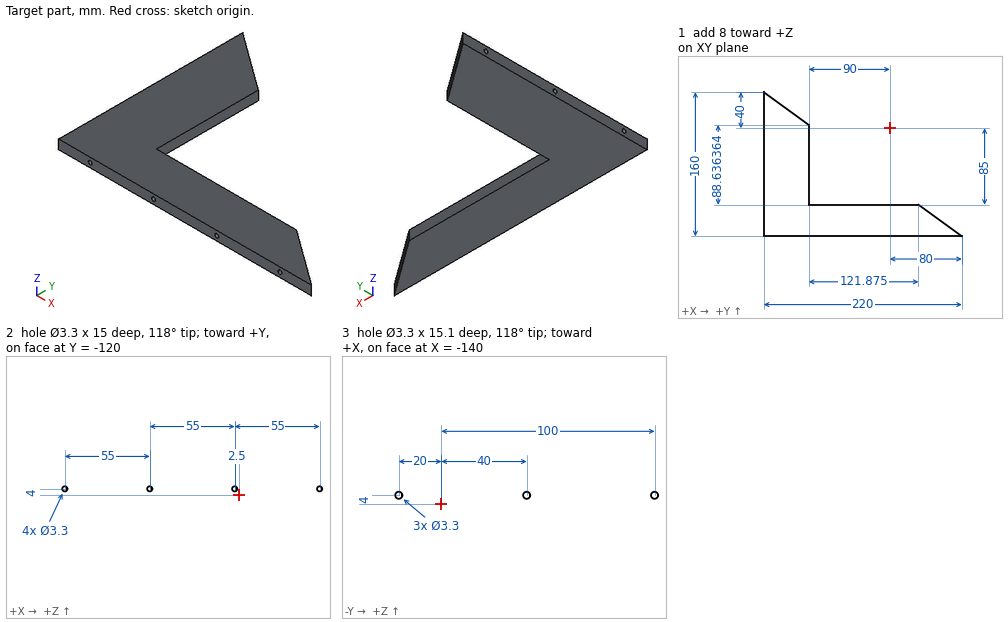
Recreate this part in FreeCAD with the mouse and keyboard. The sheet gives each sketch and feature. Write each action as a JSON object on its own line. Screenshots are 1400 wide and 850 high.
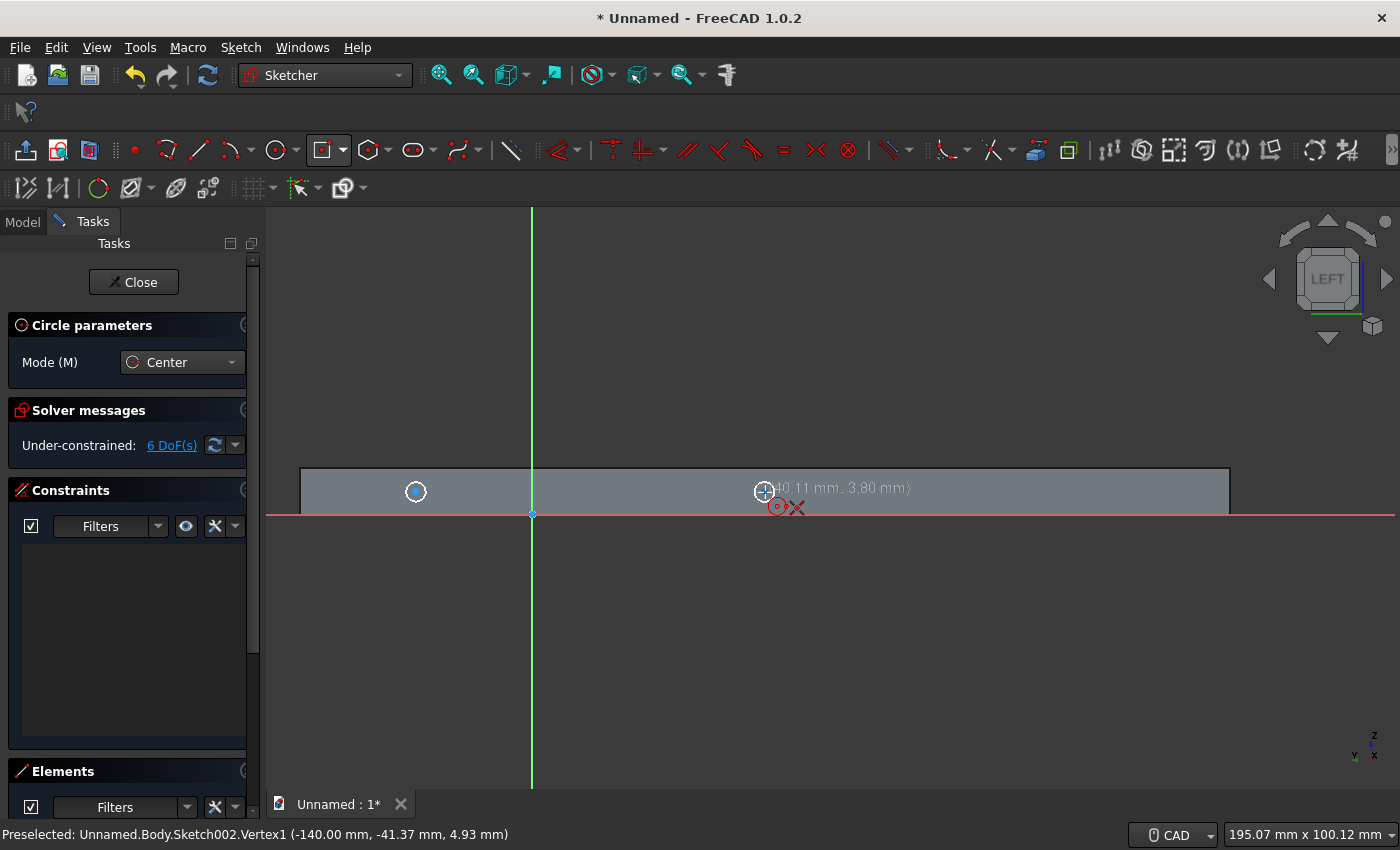
{"action": "scroll", "coordinate": [1113, 492], "scroll_direction": "up", "scroll_amount": 5}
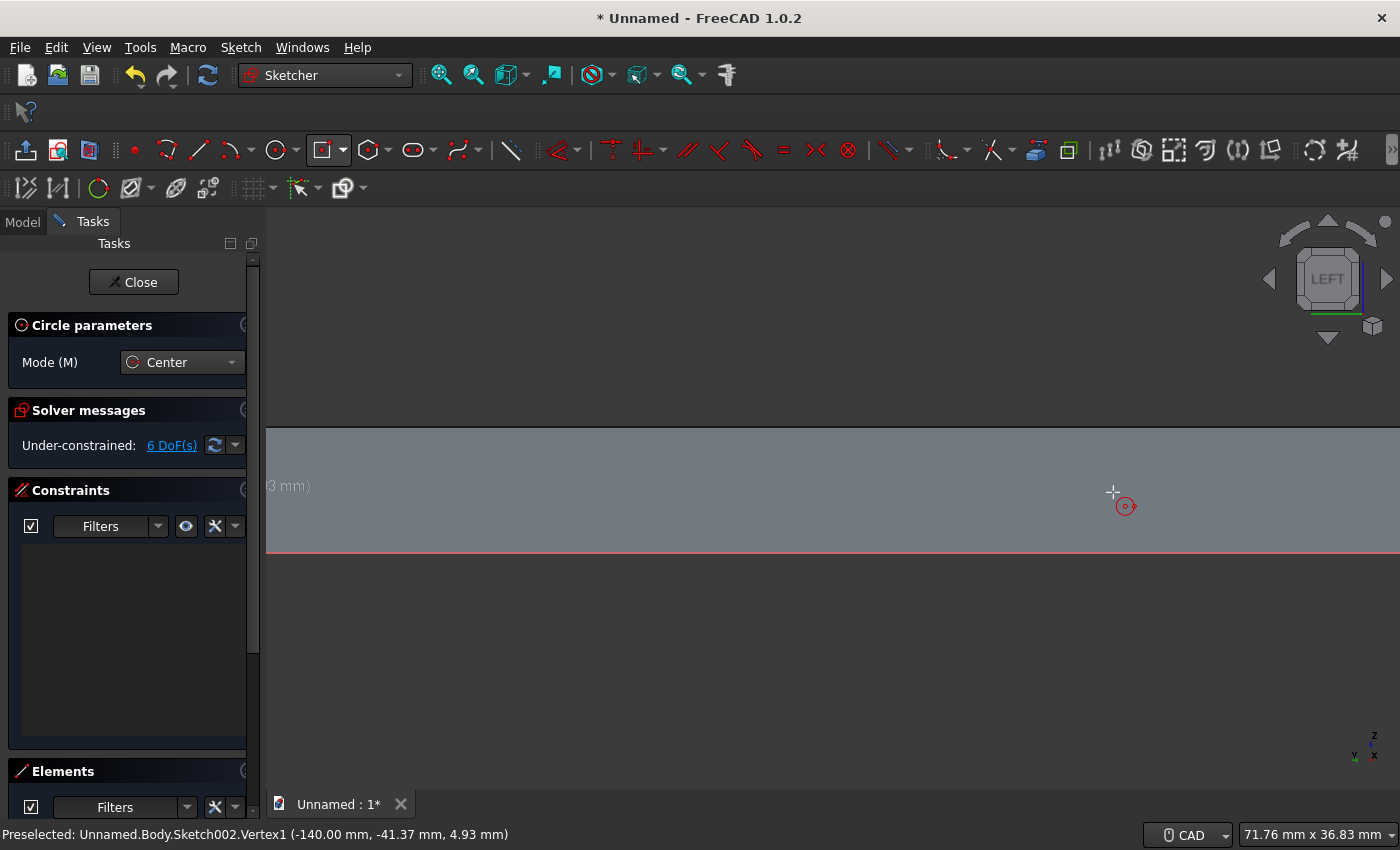
{"action": "left_click", "coordinate": [1113, 490]}
{"action": "left_click", "coordinate": [1131, 471]}
{"action": "key", "text": "Escape"}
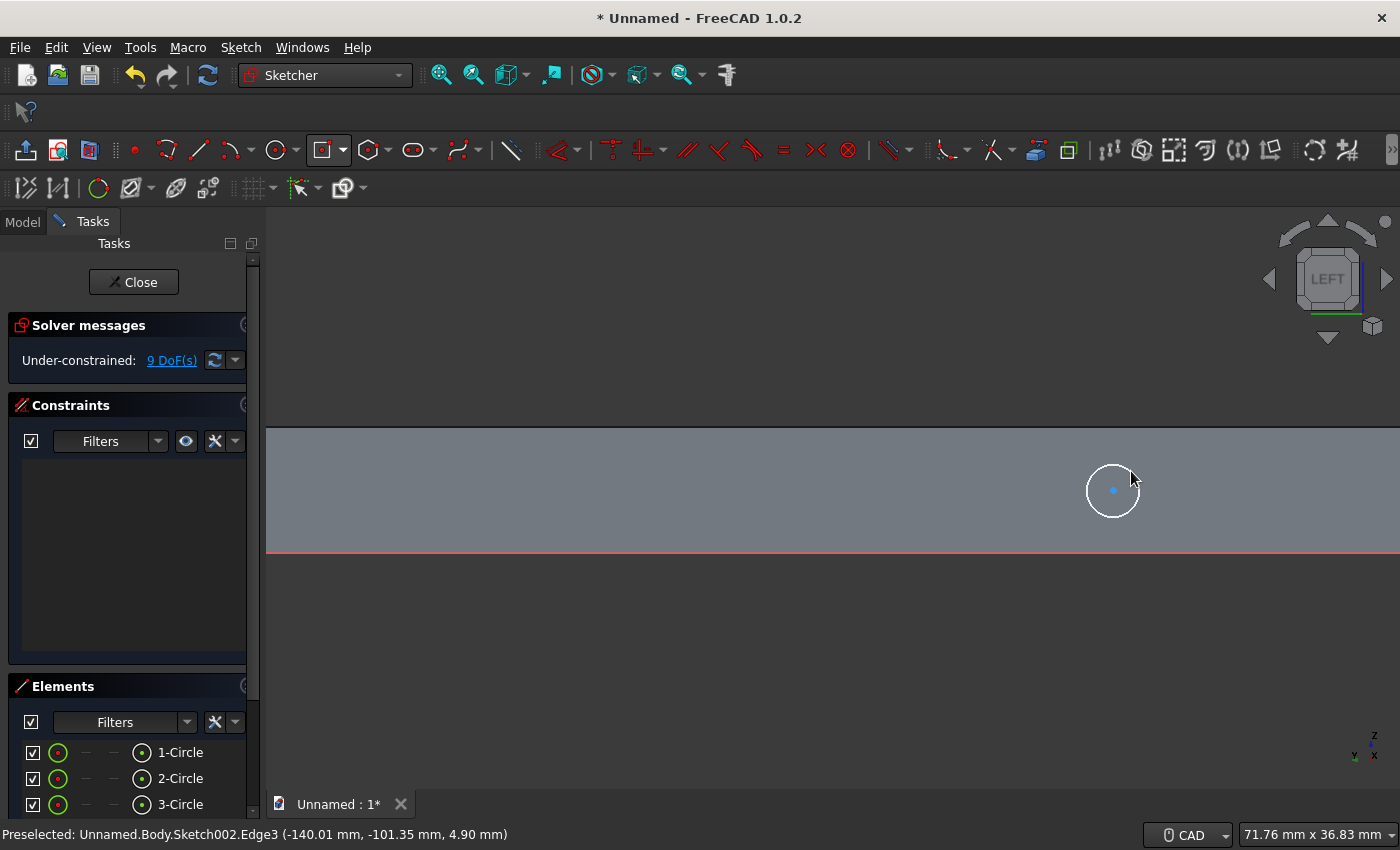
{"action": "scroll", "coordinate": [1114, 492], "scroll_direction": "down", "scroll_amount": 5}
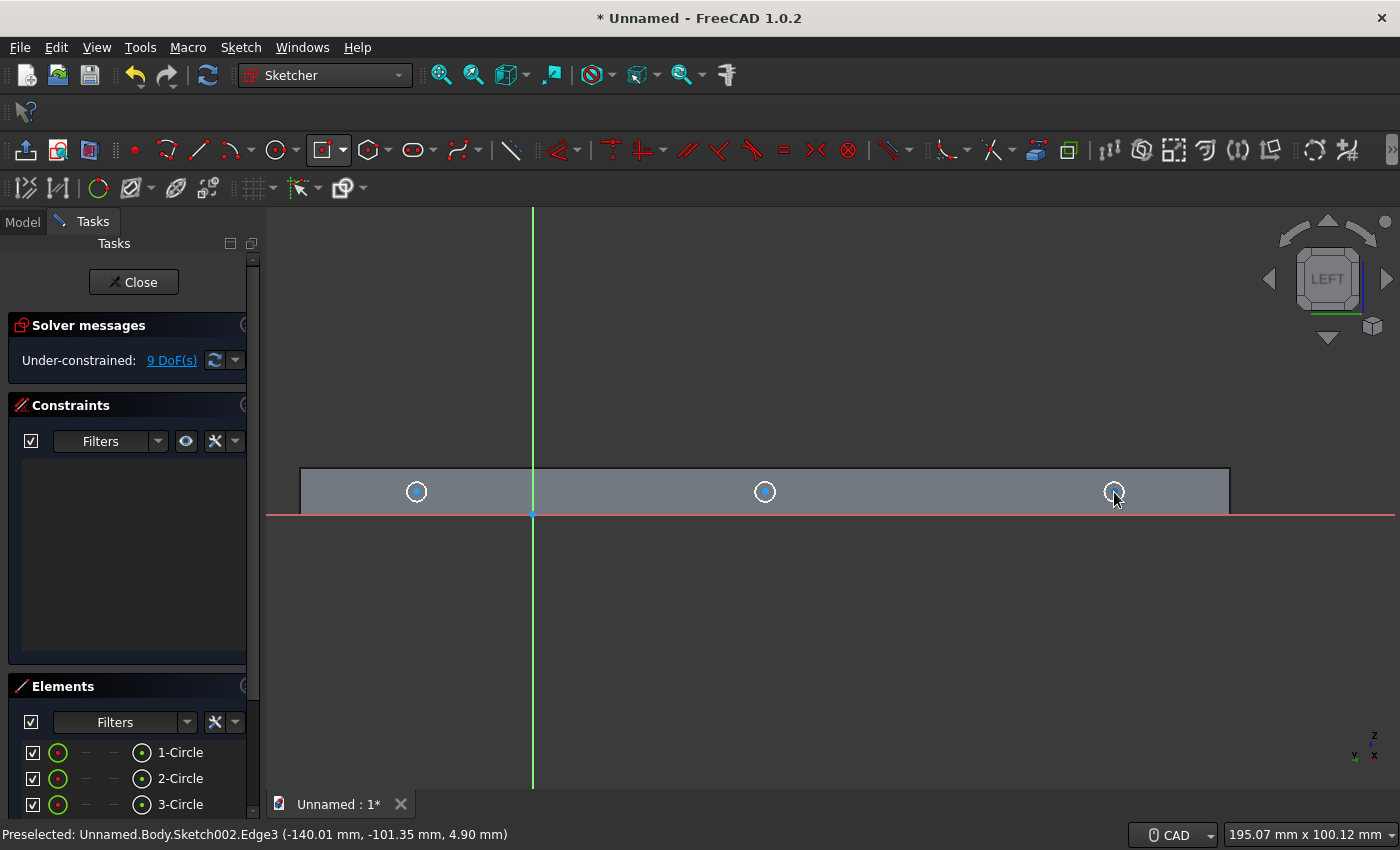
{"action": "scroll", "coordinate": [423, 485], "scroll_direction": "up", "scroll_amount": 2}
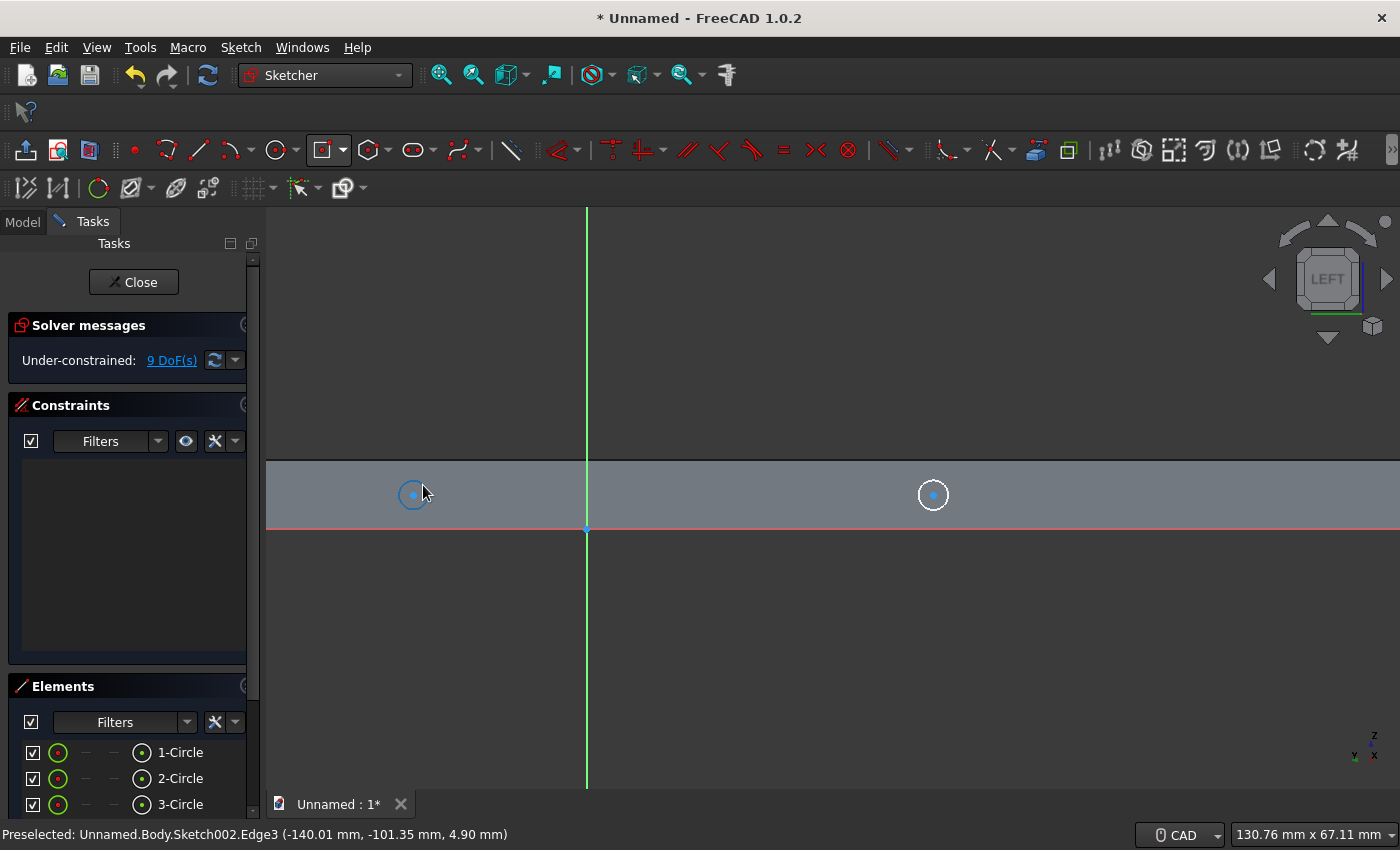
{"action": "left_click", "coordinate": [424, 485]}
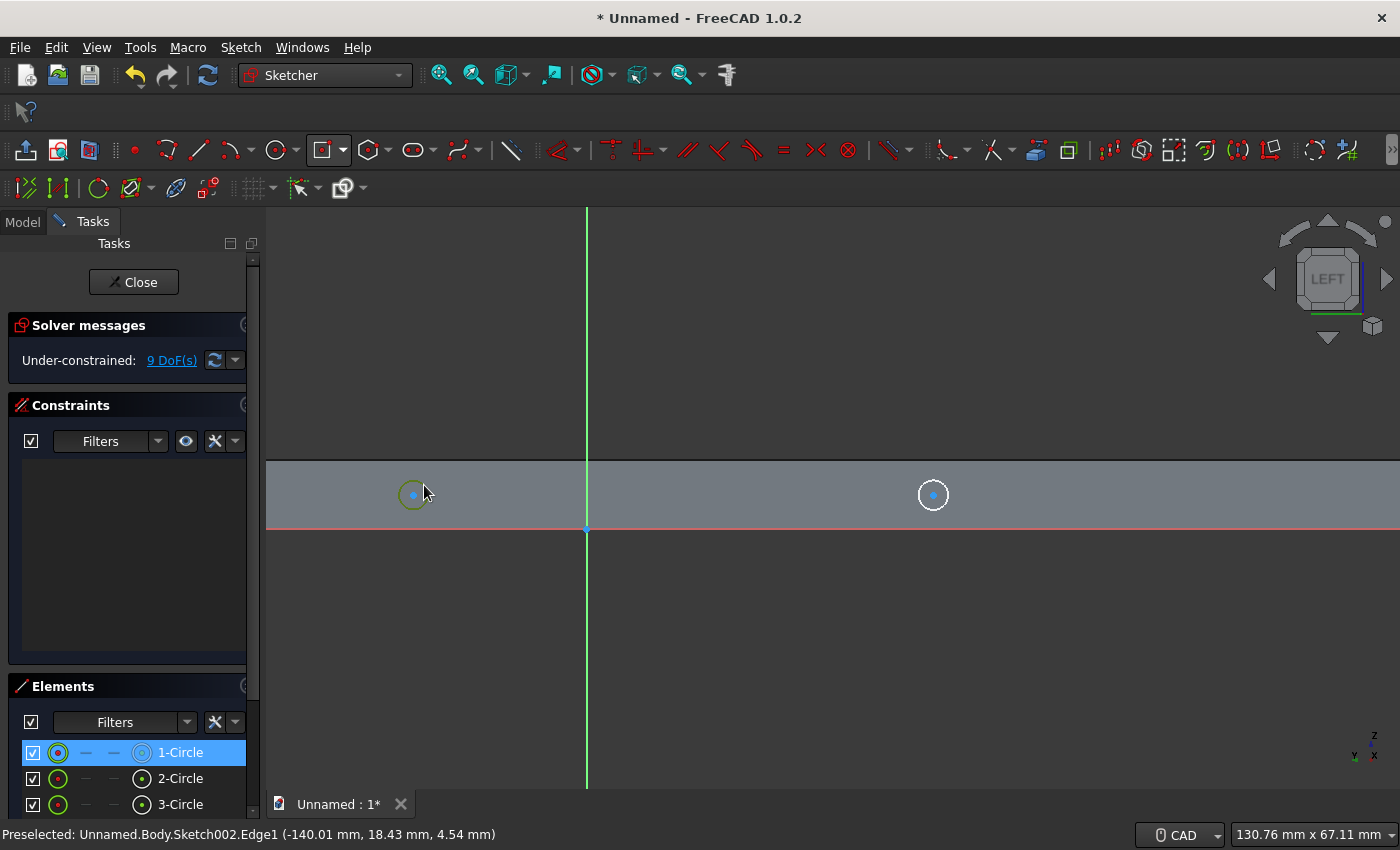
{"action": "left_click", "coordinate": [944, 485]}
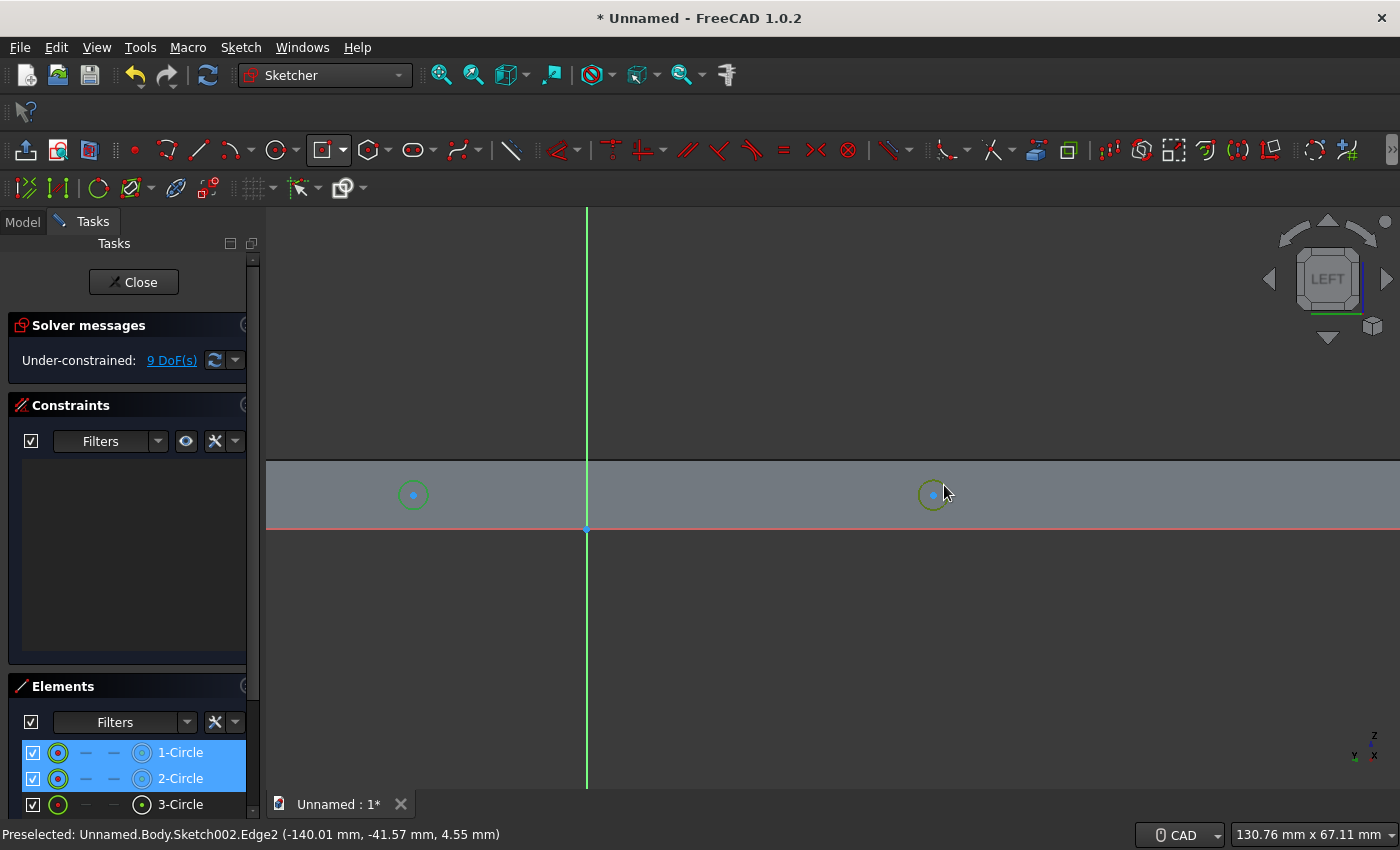
{"action": "scroll", "coordinate": [421, 484], "scroll_direction": "down", "scroll_amount": 2}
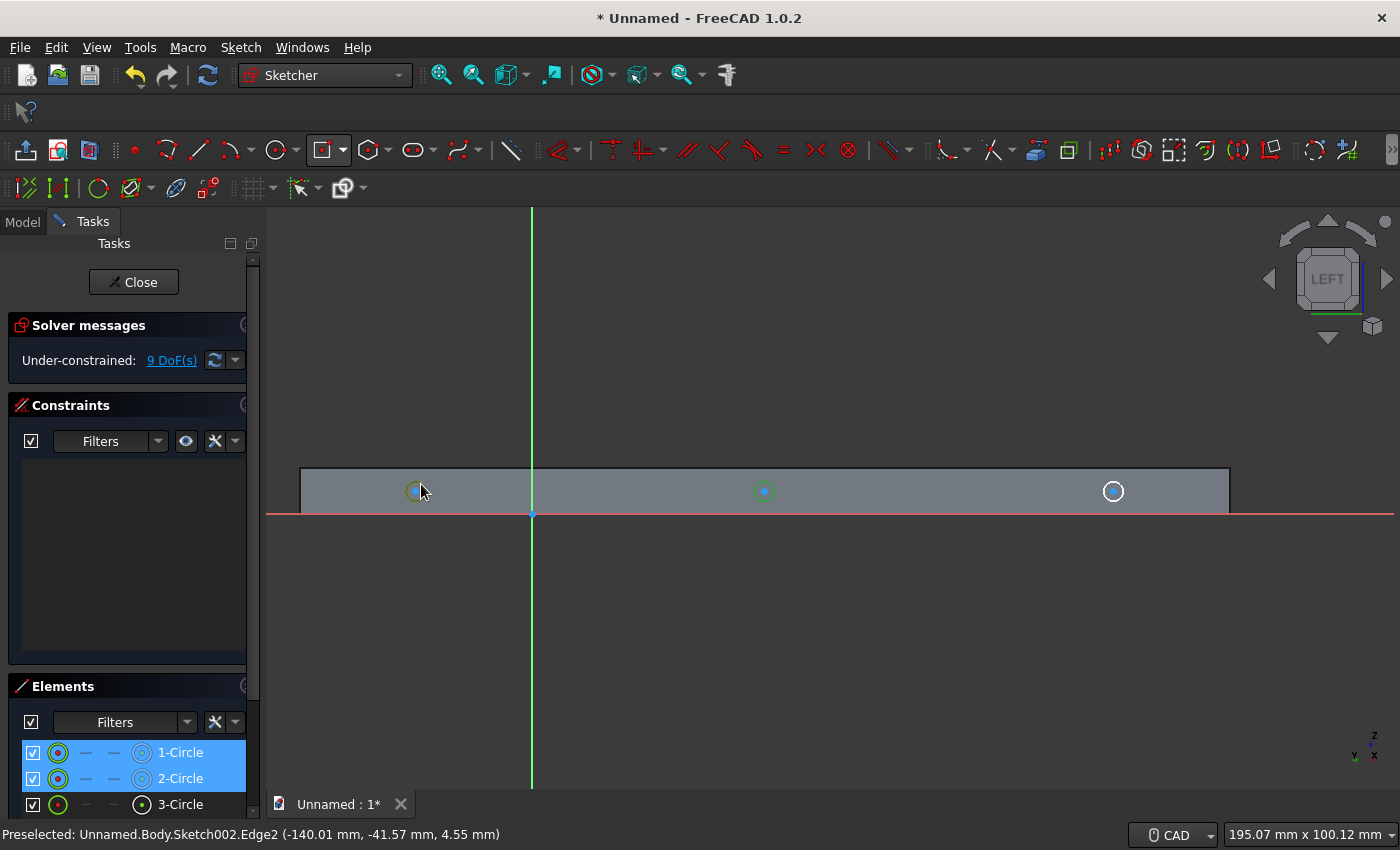
{"action": "scroll", "coordinate": [1120, 485], "scroll_direction": "up", "scroll_amount": 2}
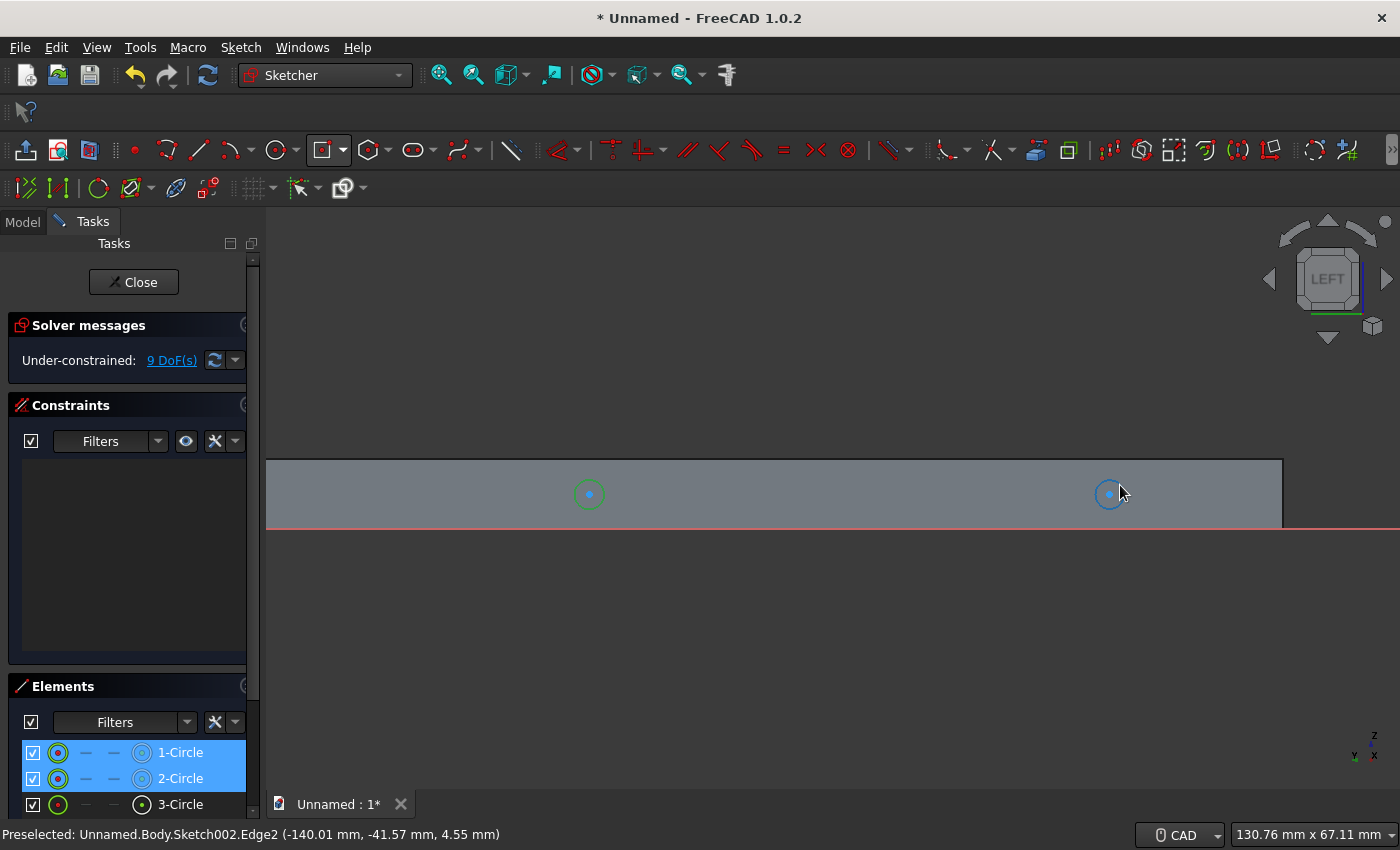
{"action": "left_click", "coordinate": [1120, 484]}